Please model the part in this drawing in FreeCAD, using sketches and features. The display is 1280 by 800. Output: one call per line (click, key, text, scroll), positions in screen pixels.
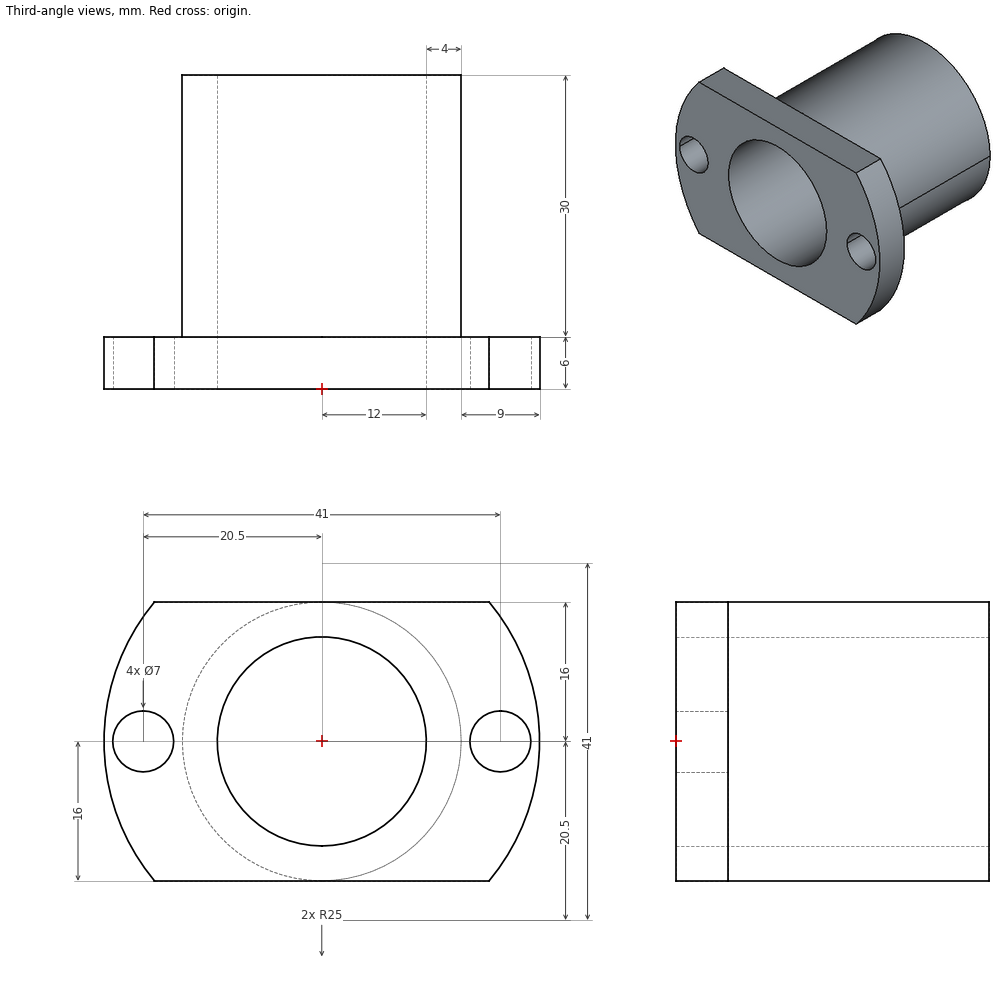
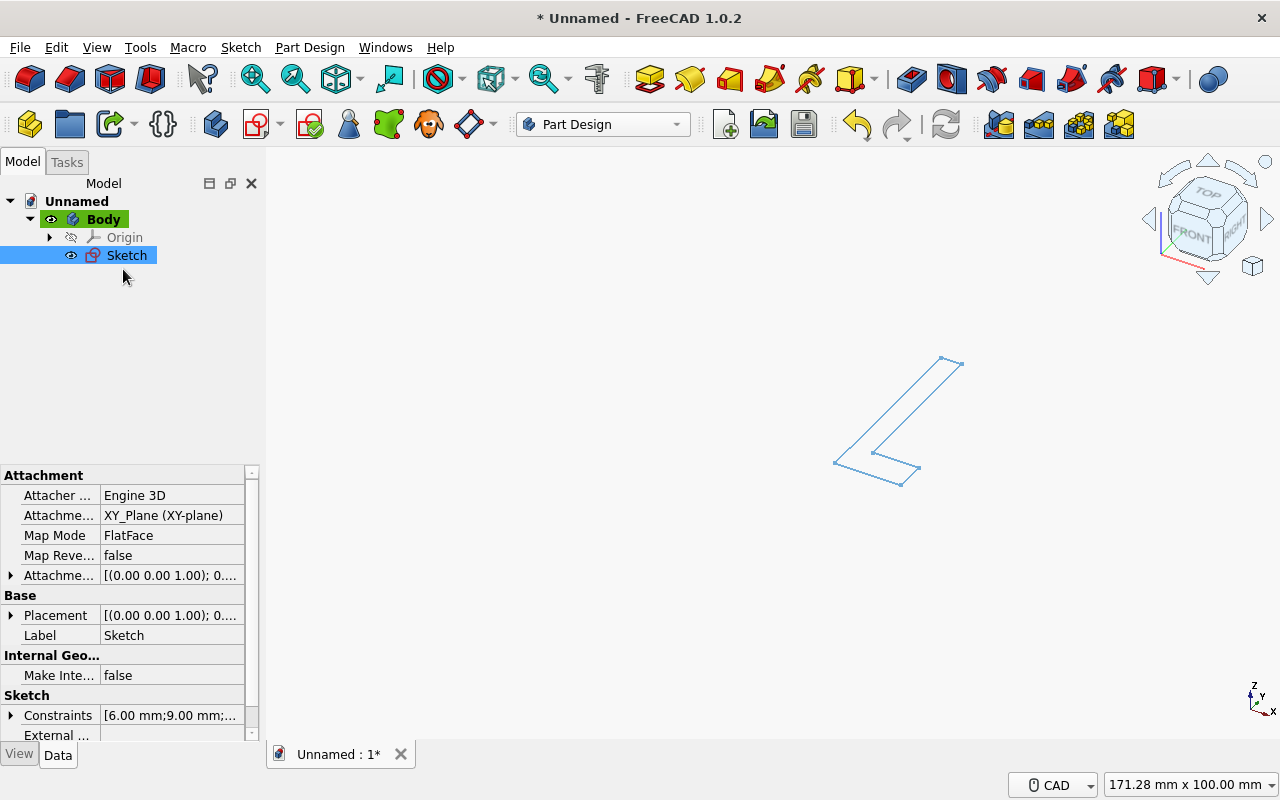
click(690, 80)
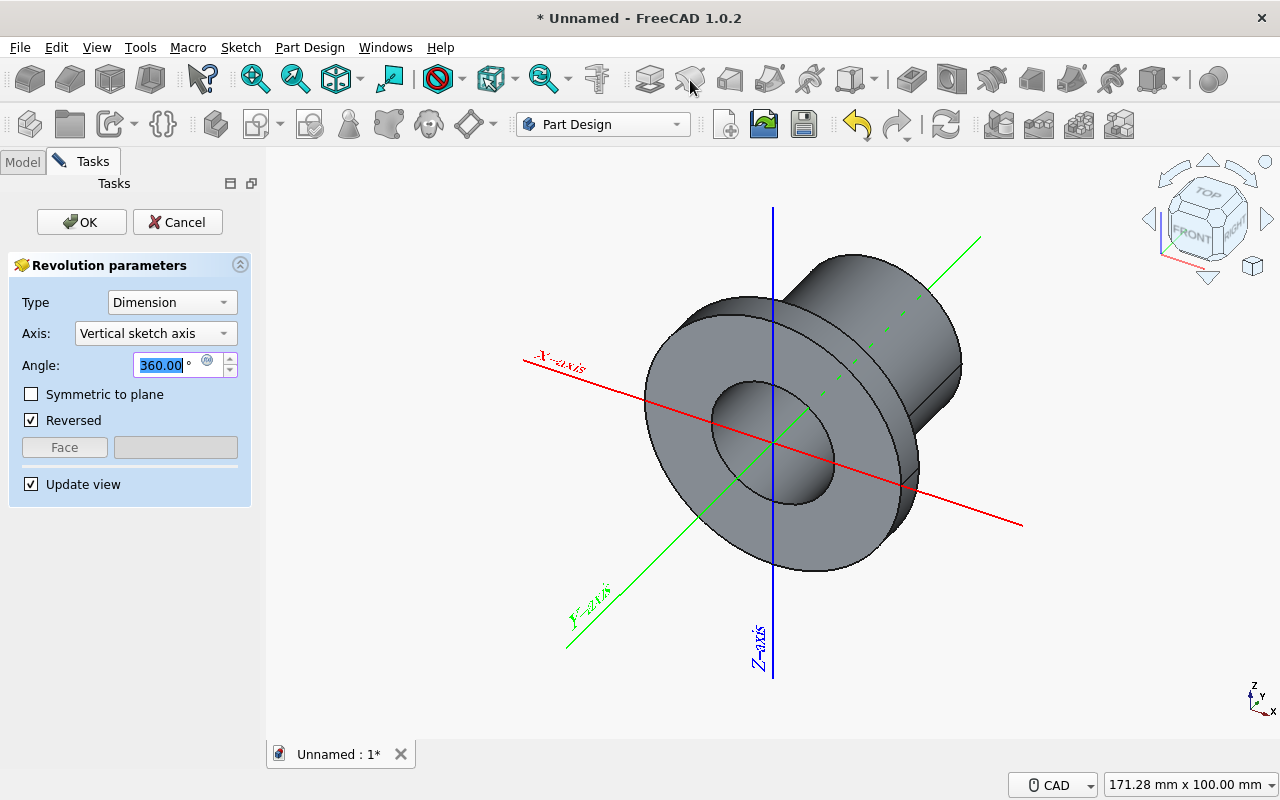
click(82, 222)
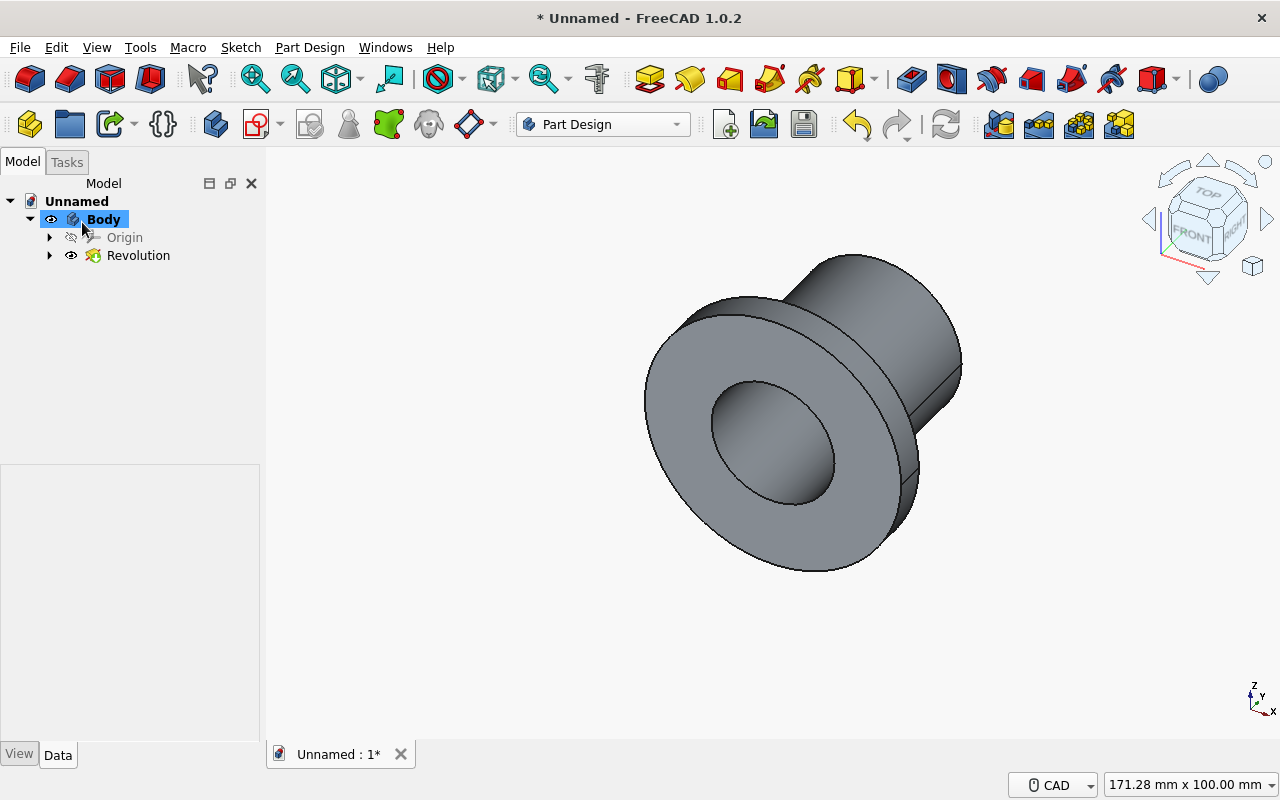
key(4)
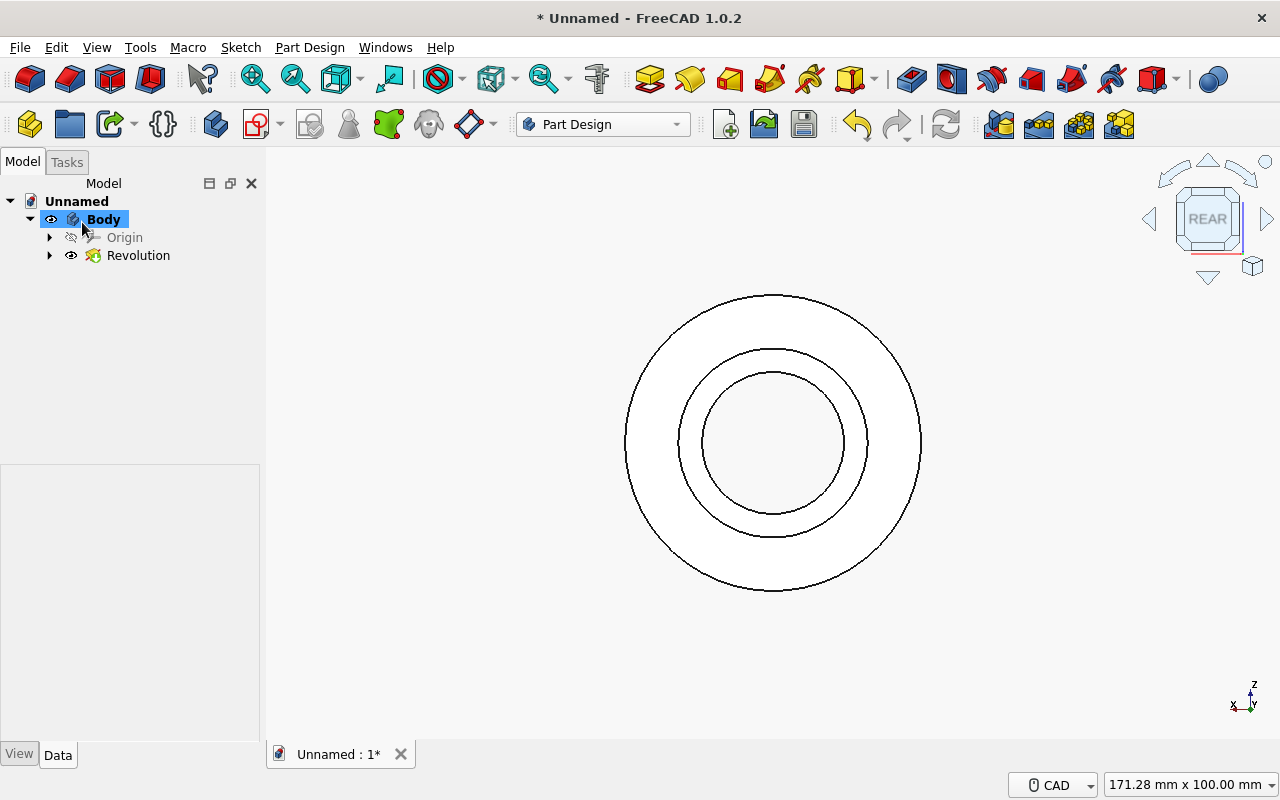
click(688, 527)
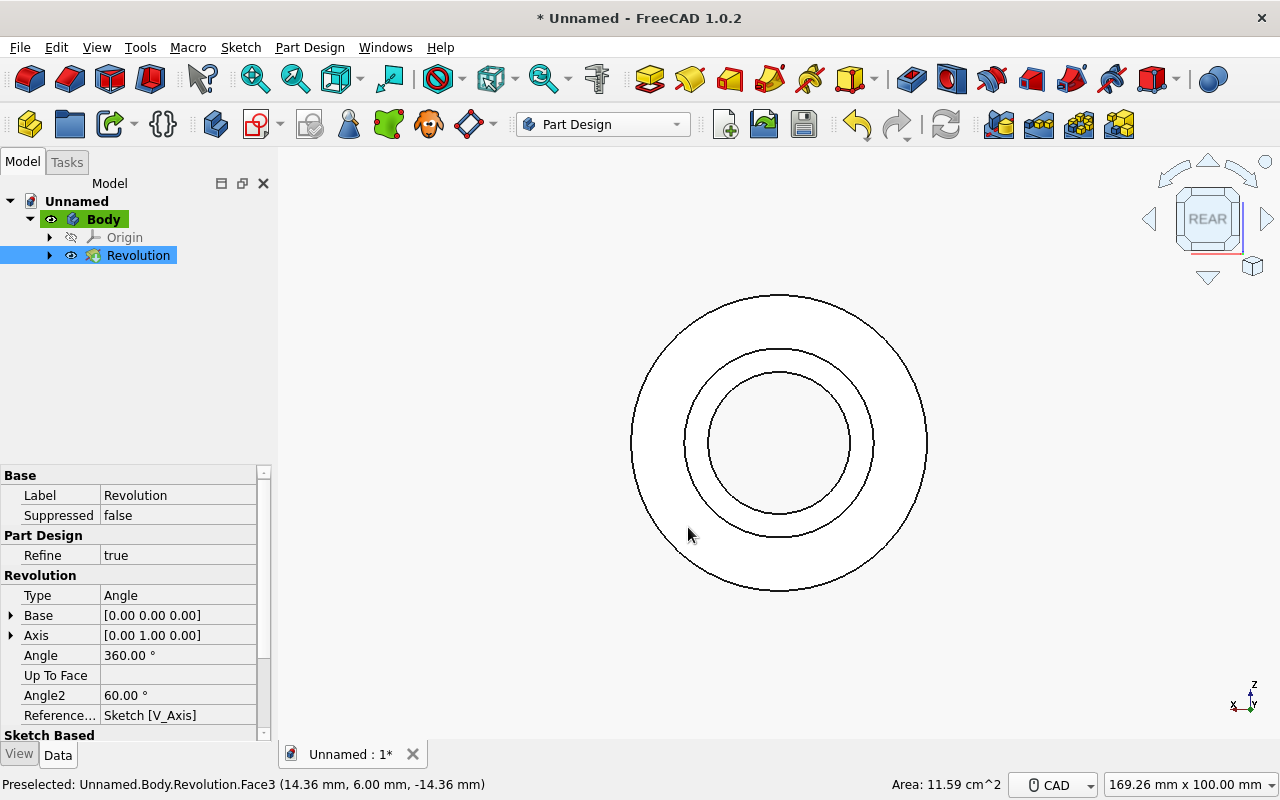
click(256, 124)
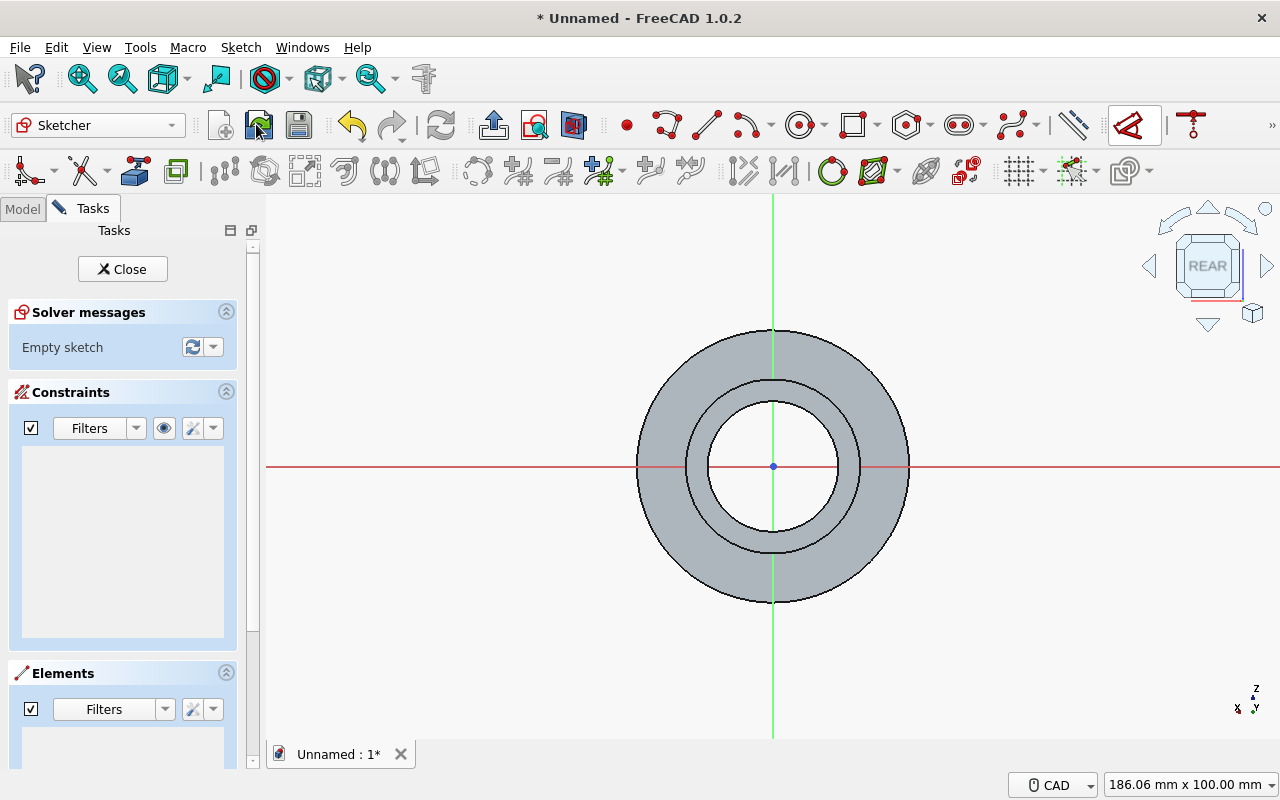
click(800, 126)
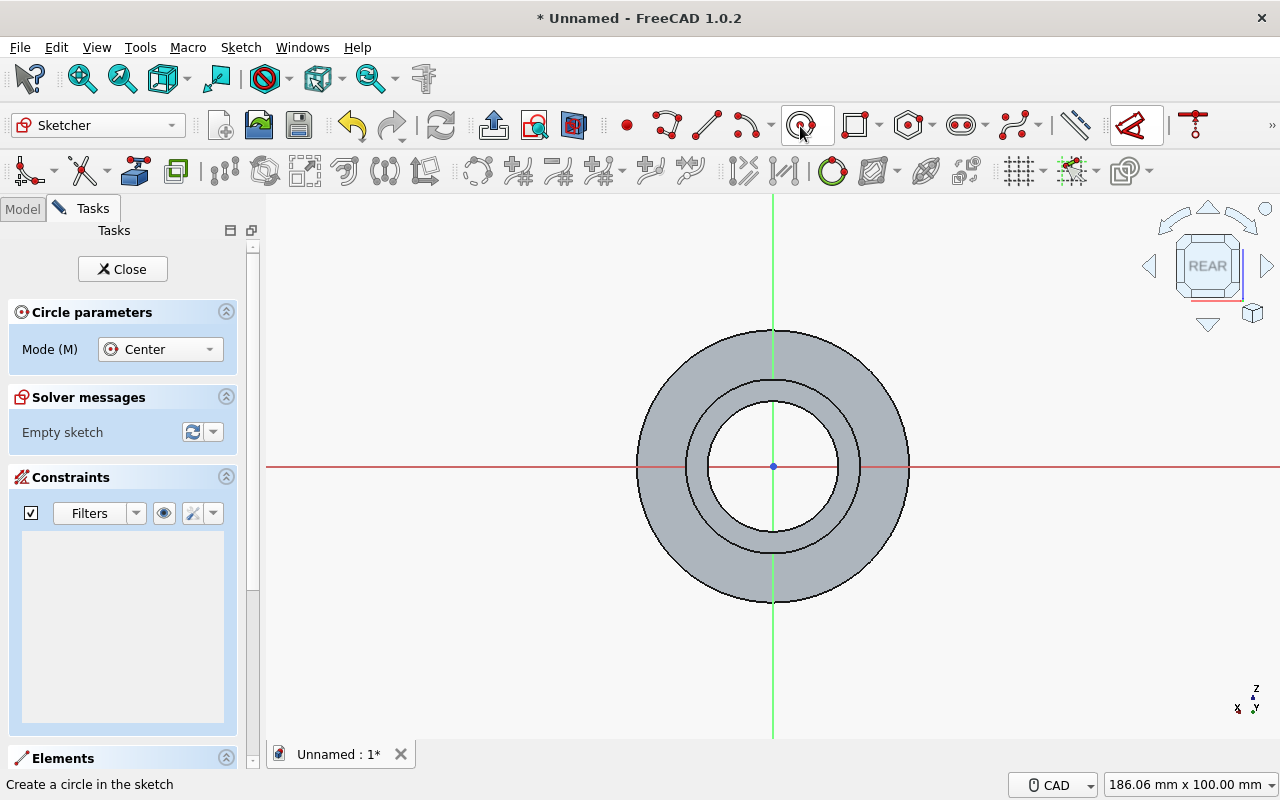
click(885, 466)
move(891, 449)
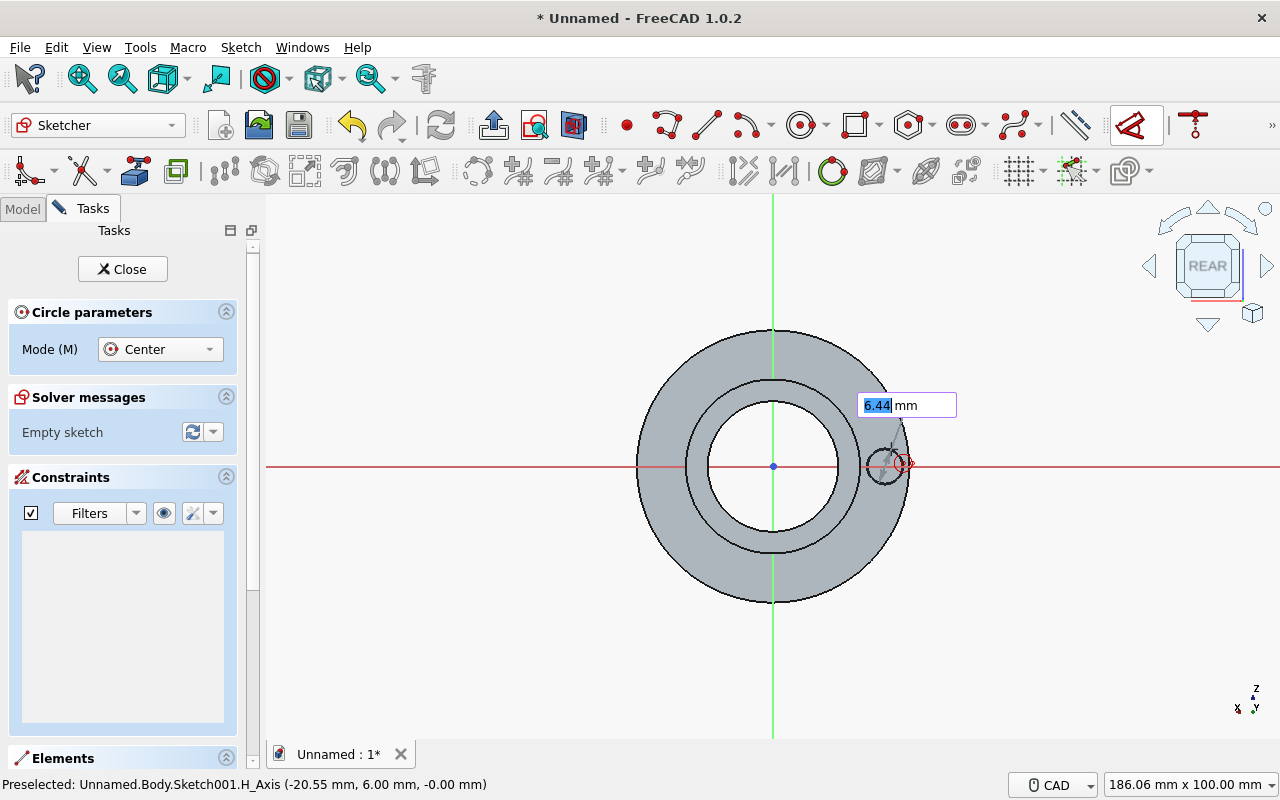
text(7)
key(Return)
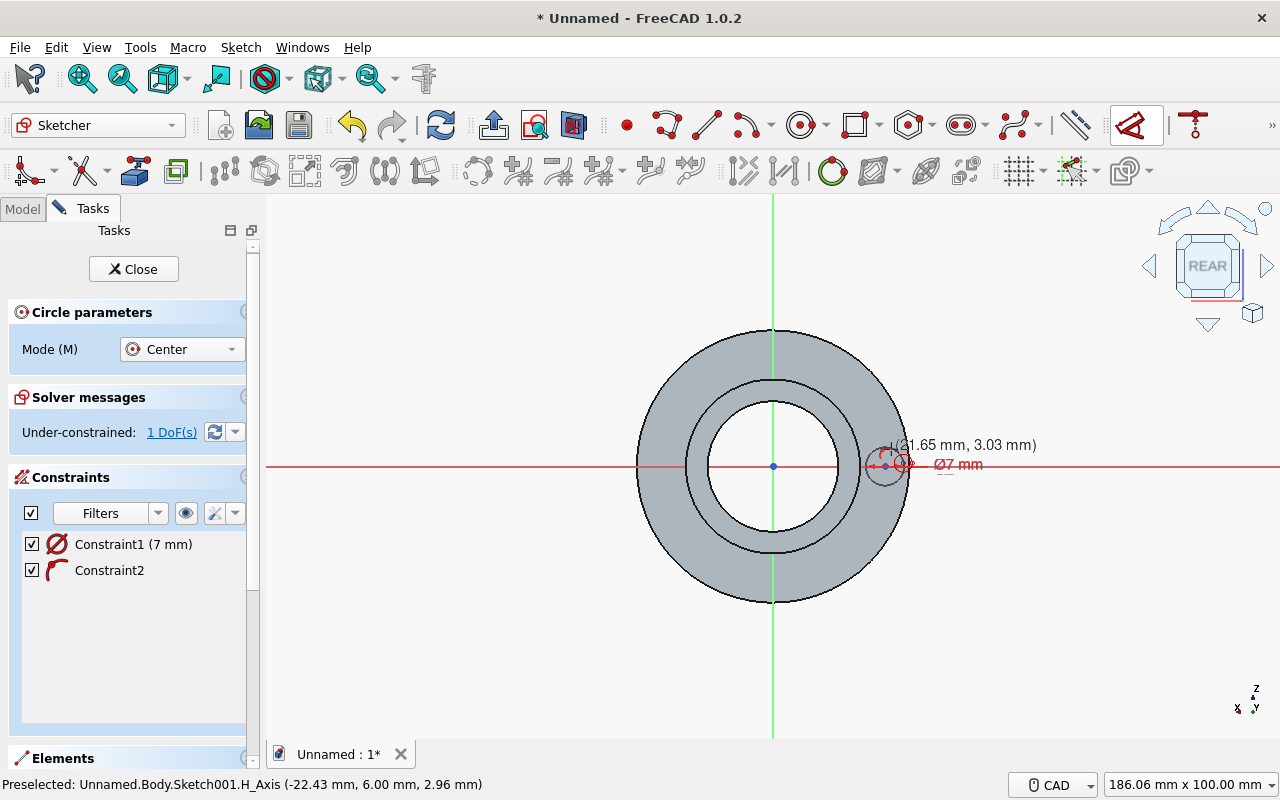
click(773, 578)
move(791, 572)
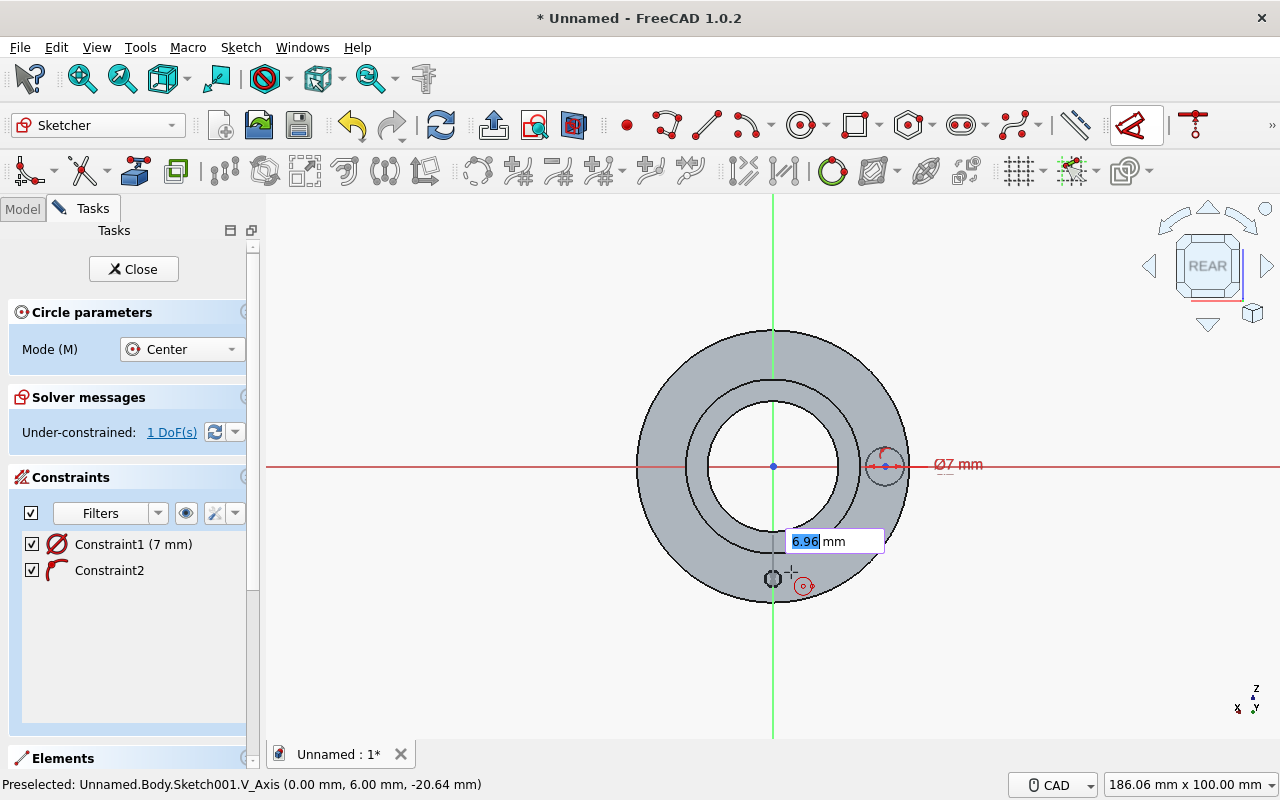
text(7)
key(Return)